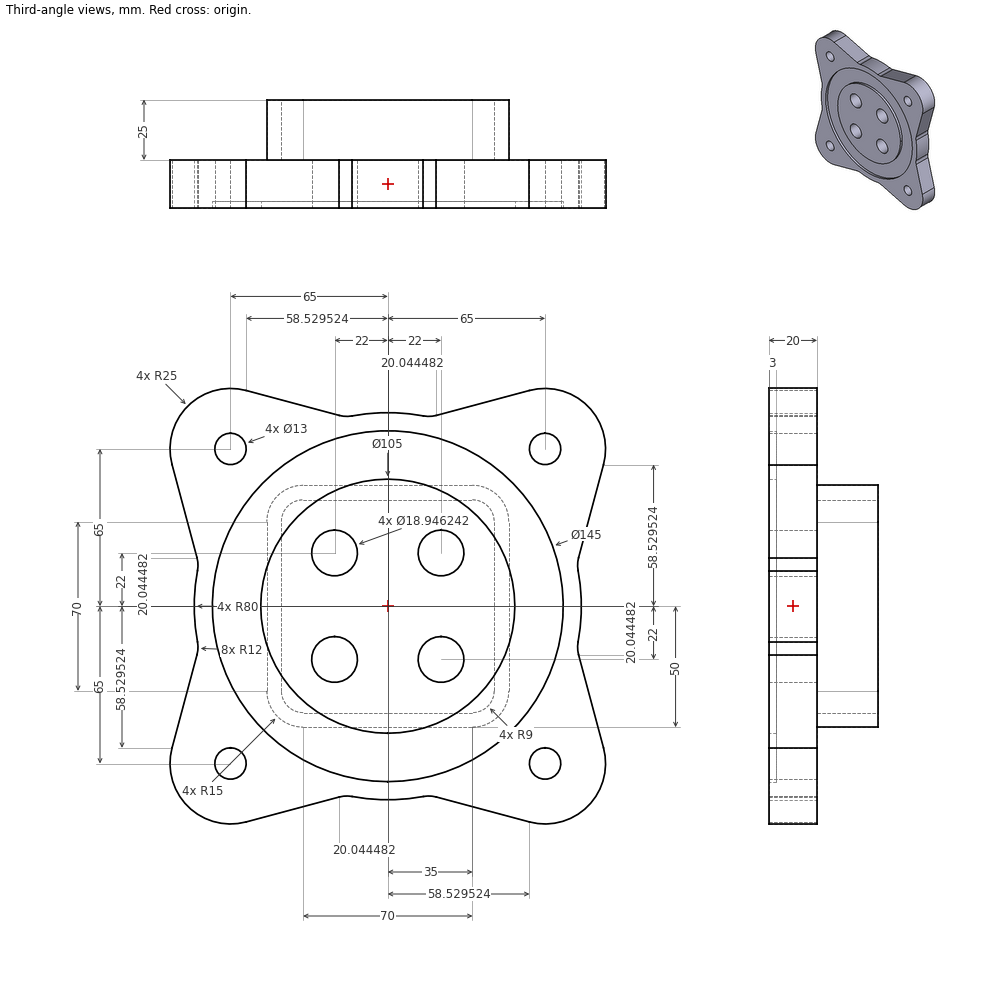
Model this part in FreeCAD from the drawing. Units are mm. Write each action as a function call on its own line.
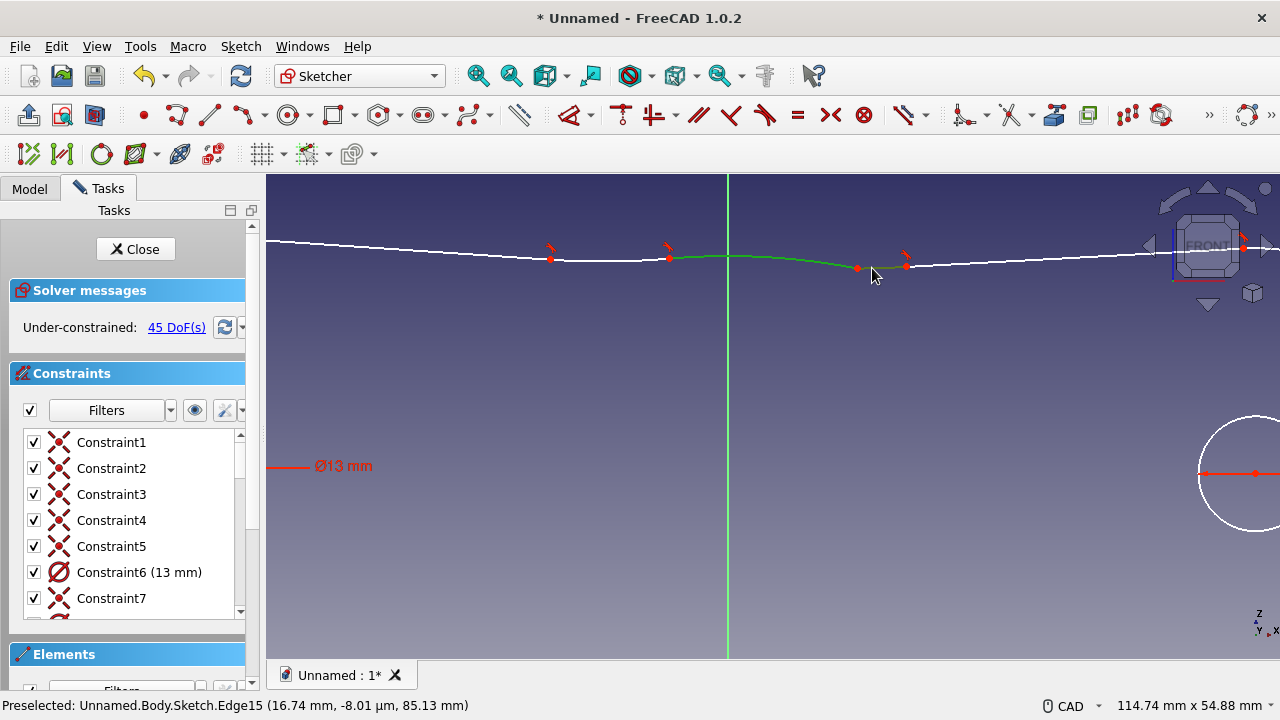
key(t)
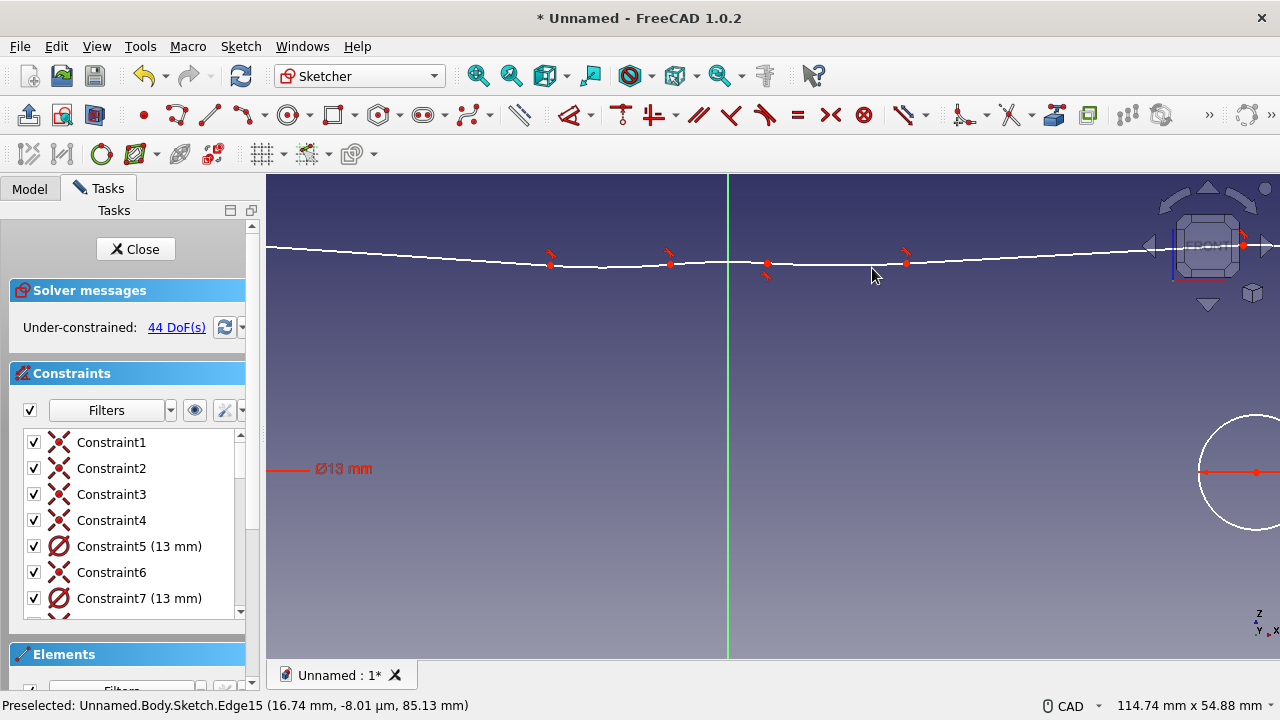
scroll(698, 264, down, 8)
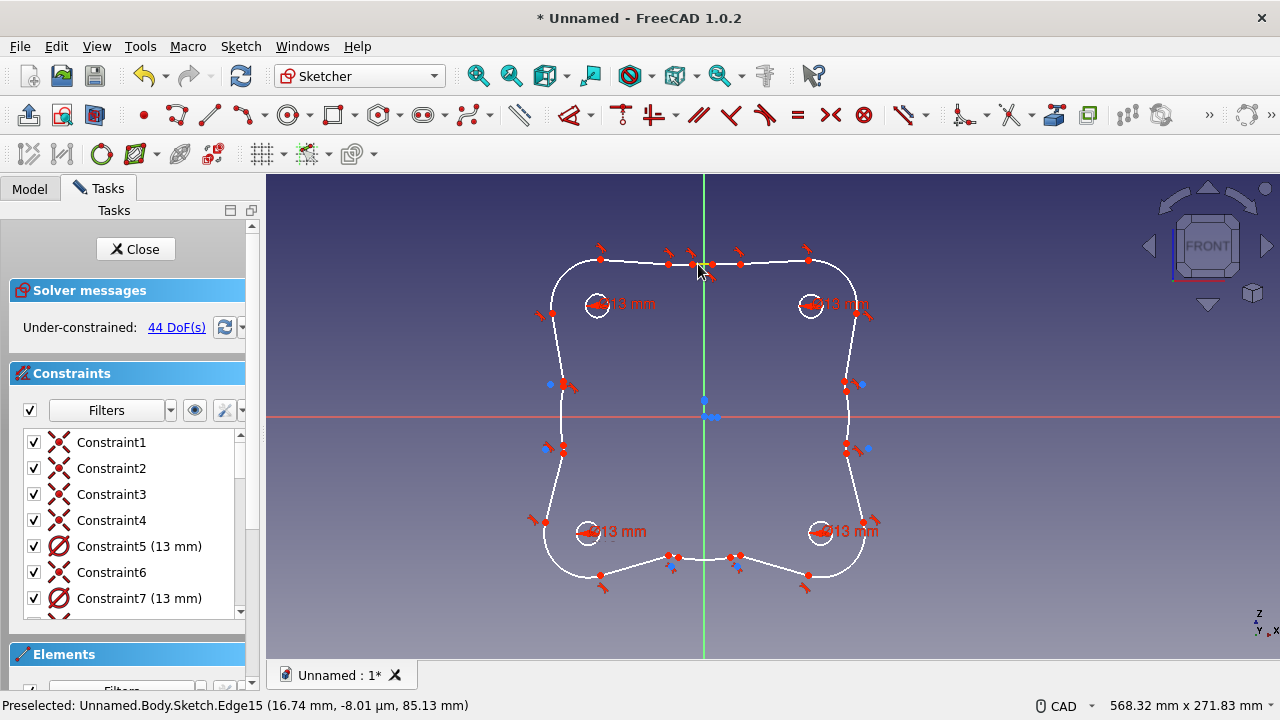
scroll(845, 385, up, 8)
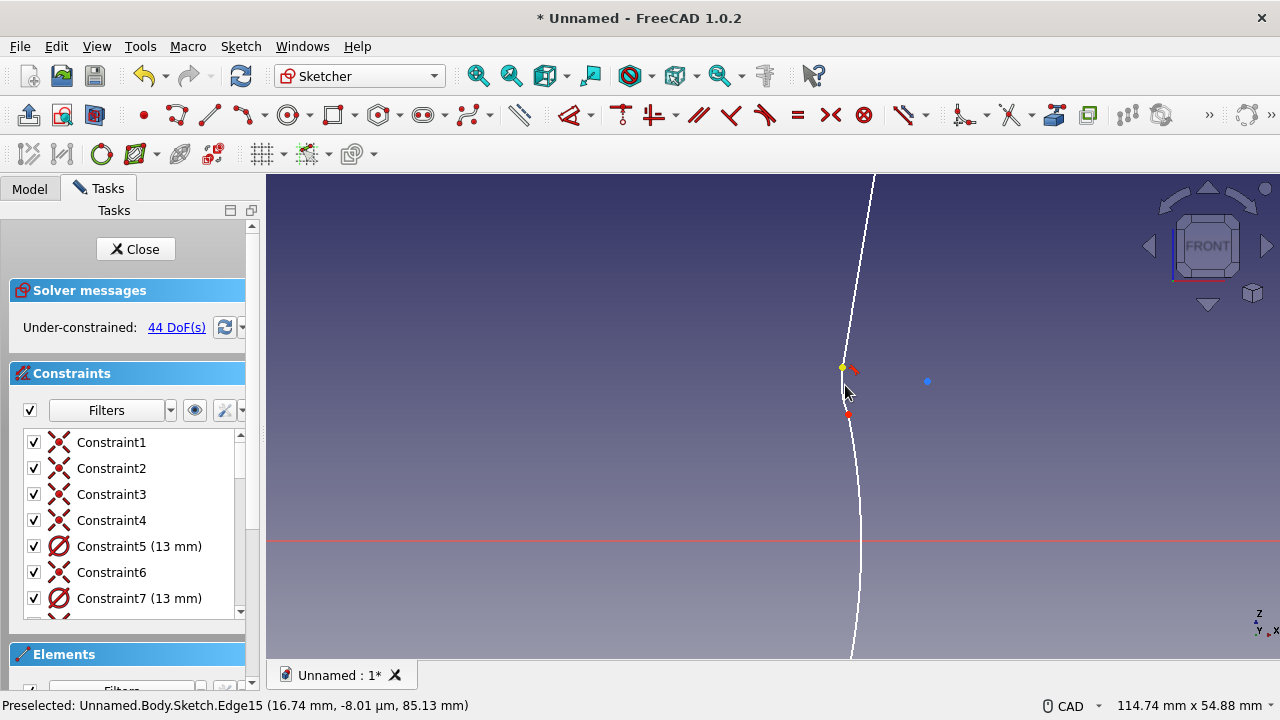
click(842, 382)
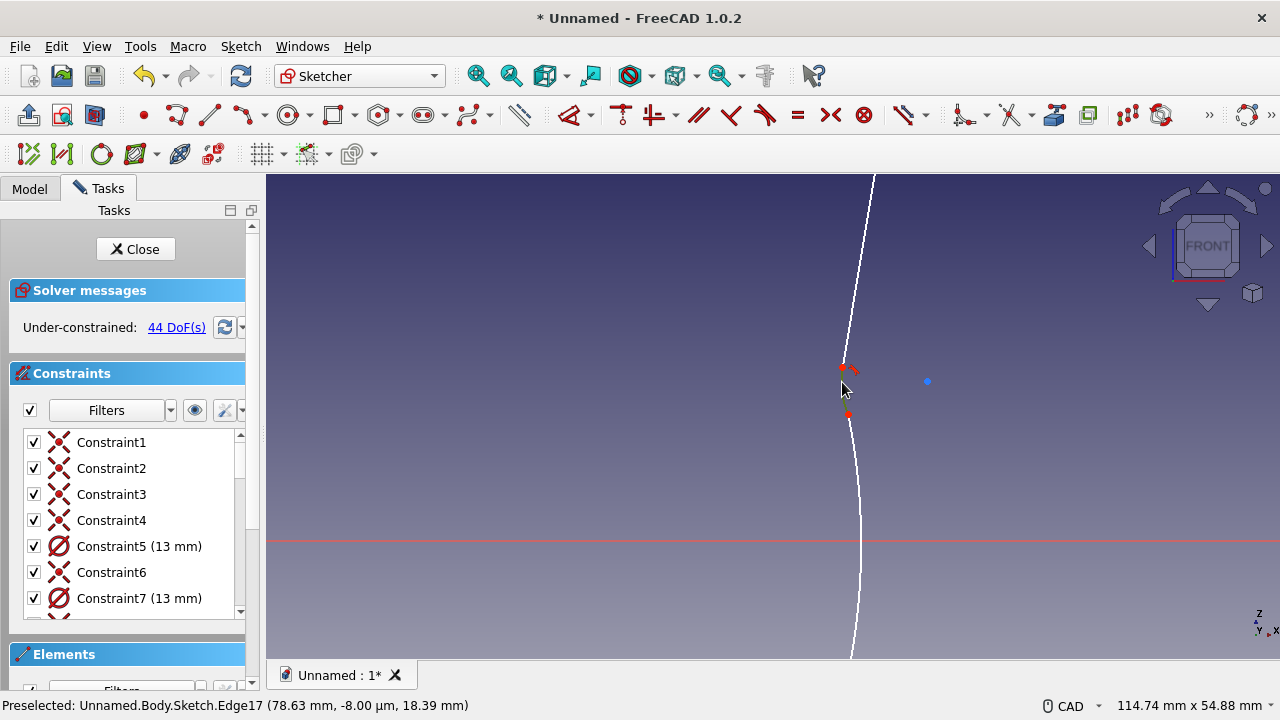
scroll(846, 385, down, 8)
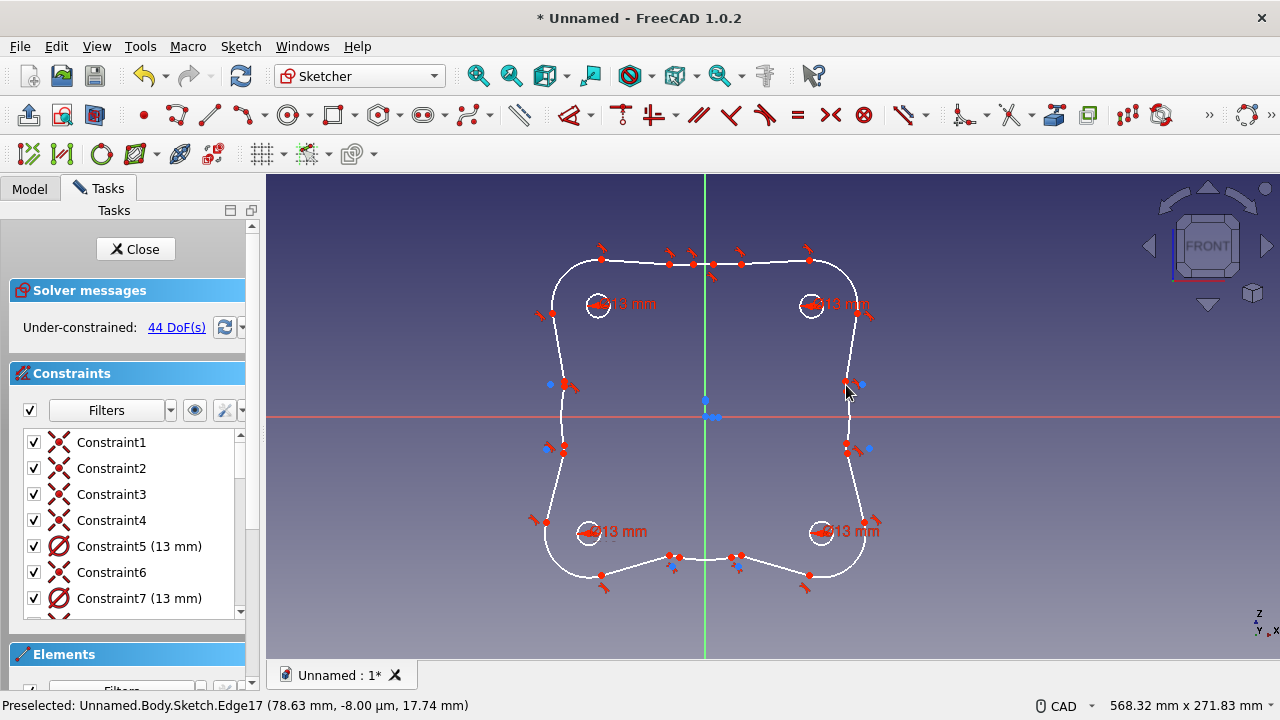
scroll(849, 428, up, 2)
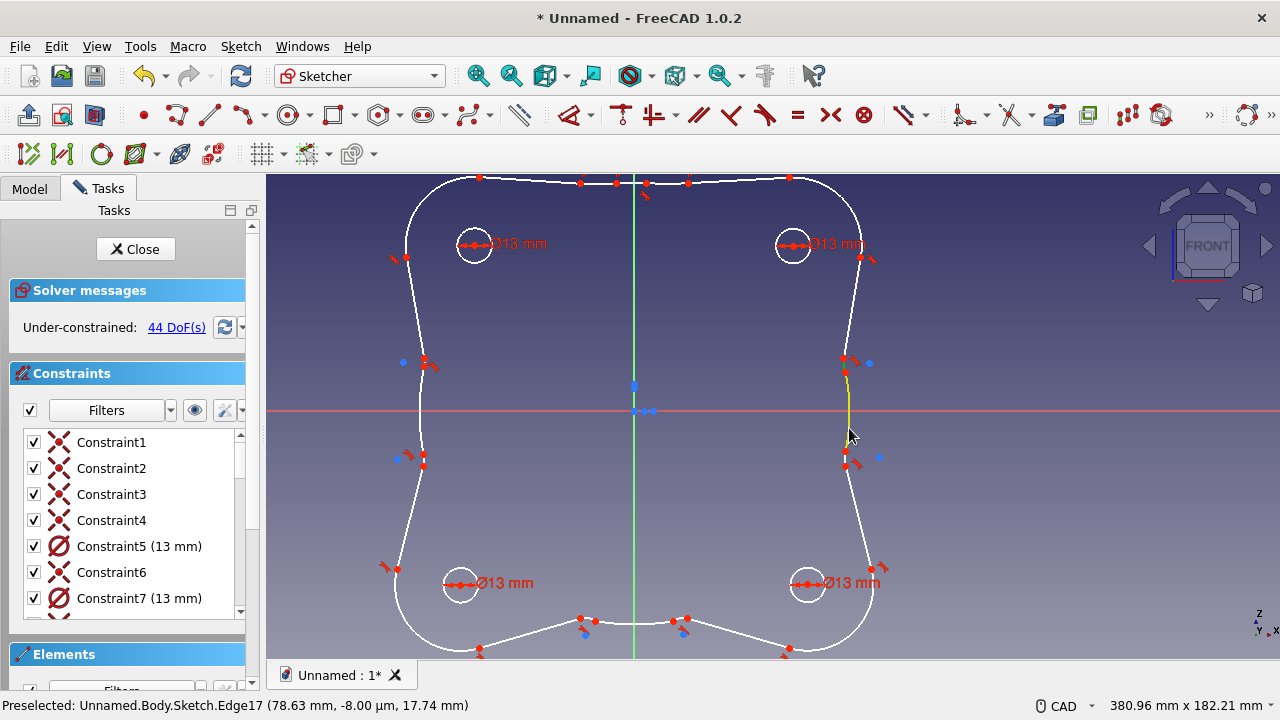
click(849, 428)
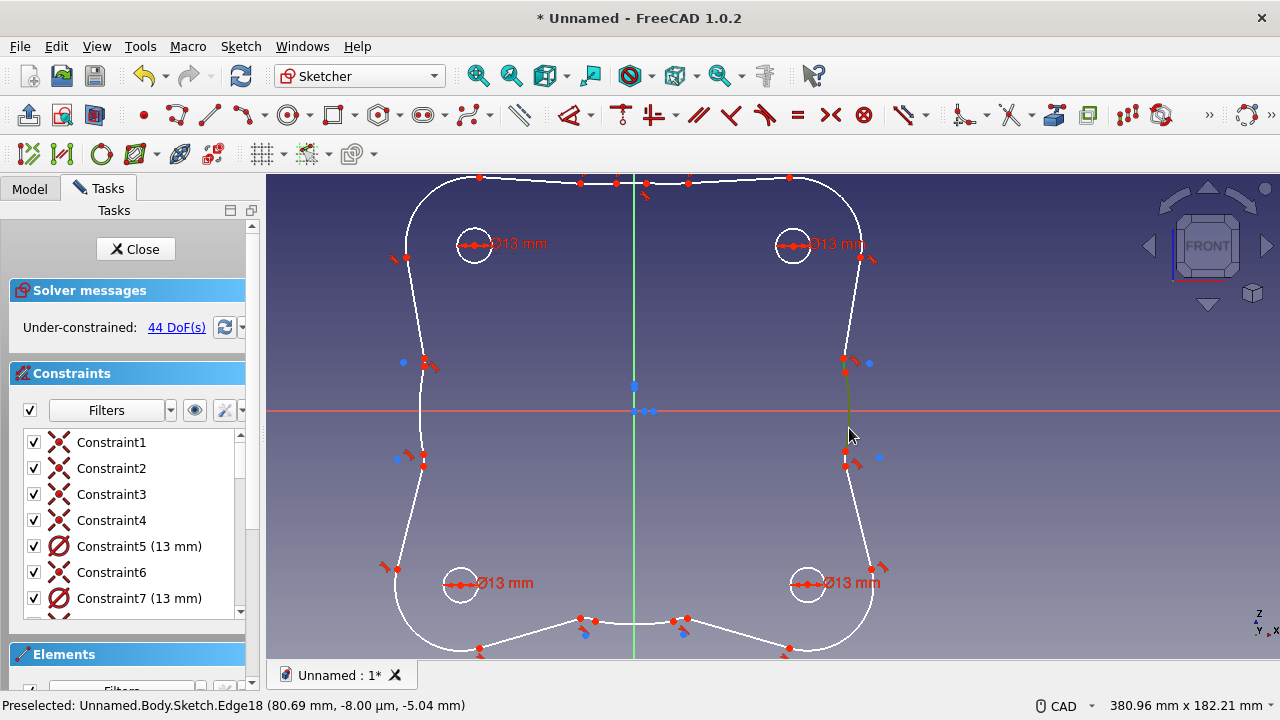
click(765, 116)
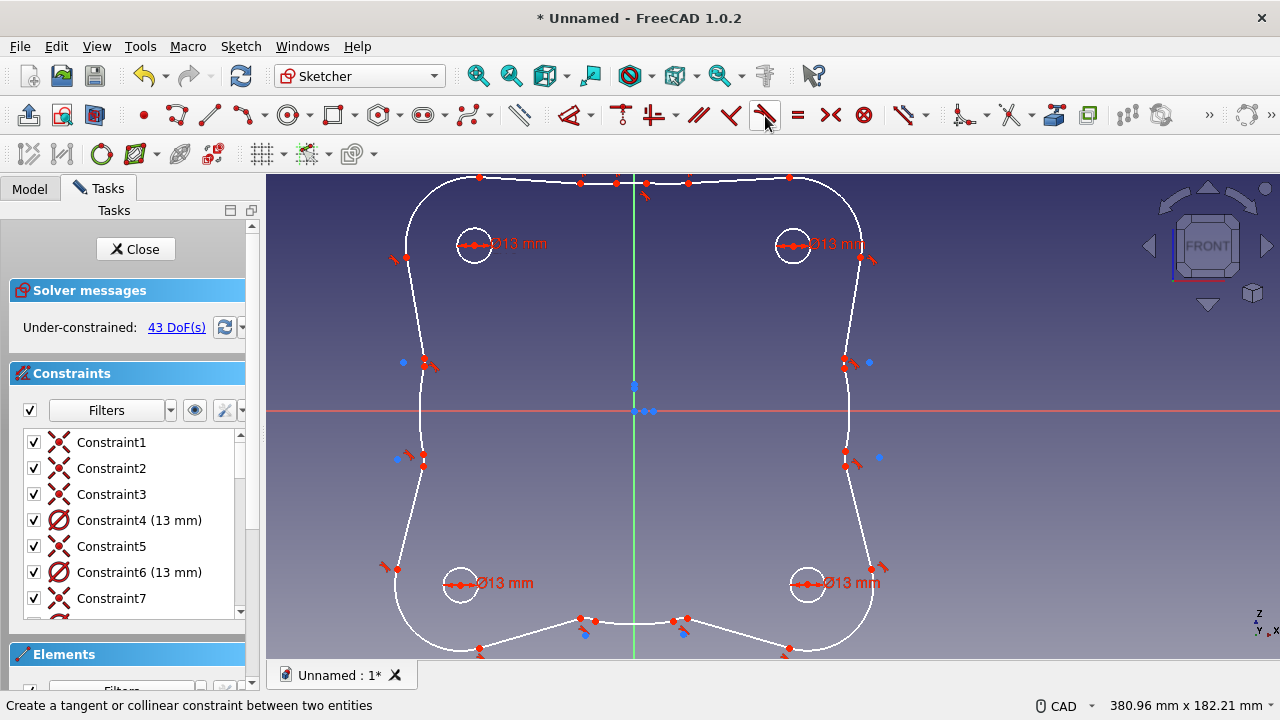
click(849, 426)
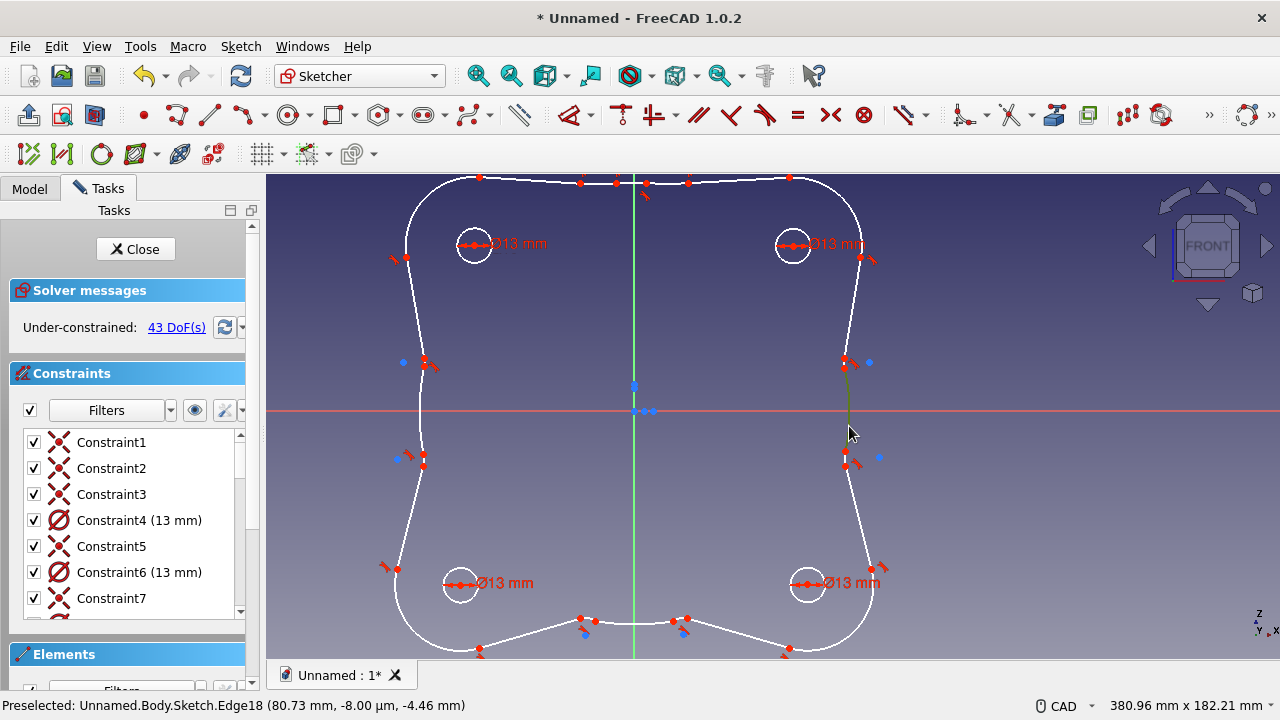
scroll(845, 459, up, 3)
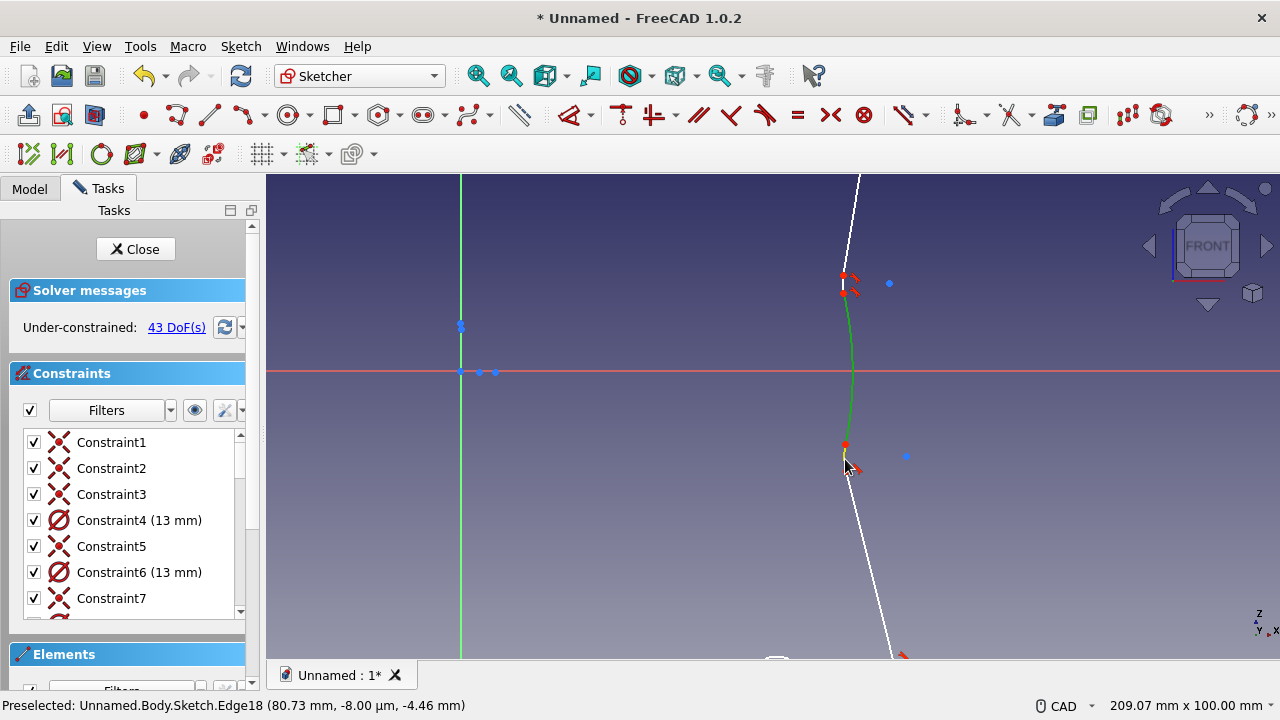
click(844, 458)